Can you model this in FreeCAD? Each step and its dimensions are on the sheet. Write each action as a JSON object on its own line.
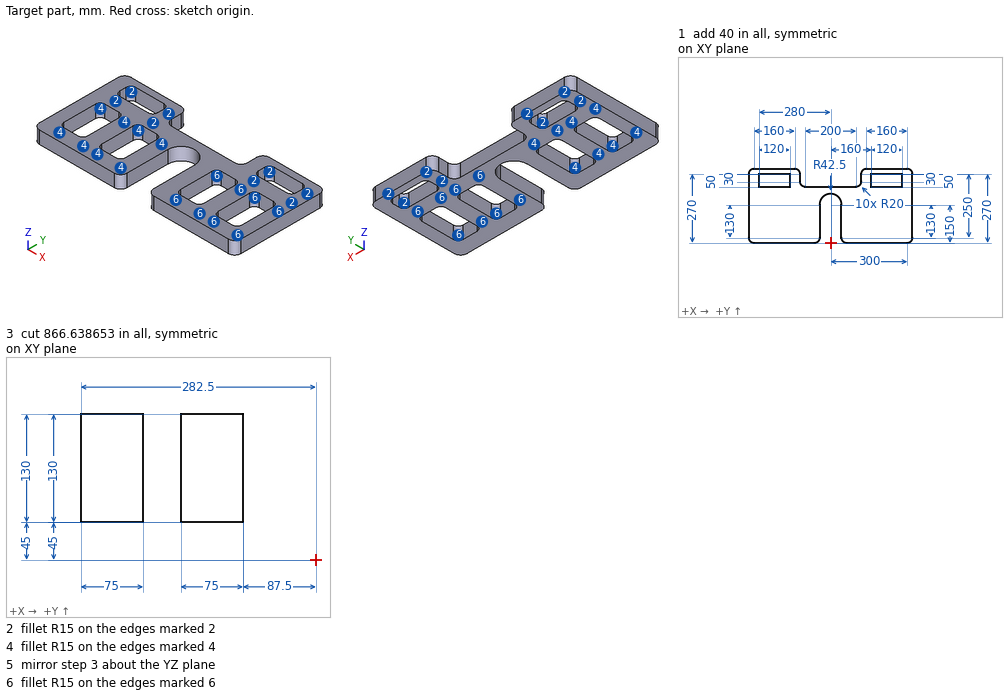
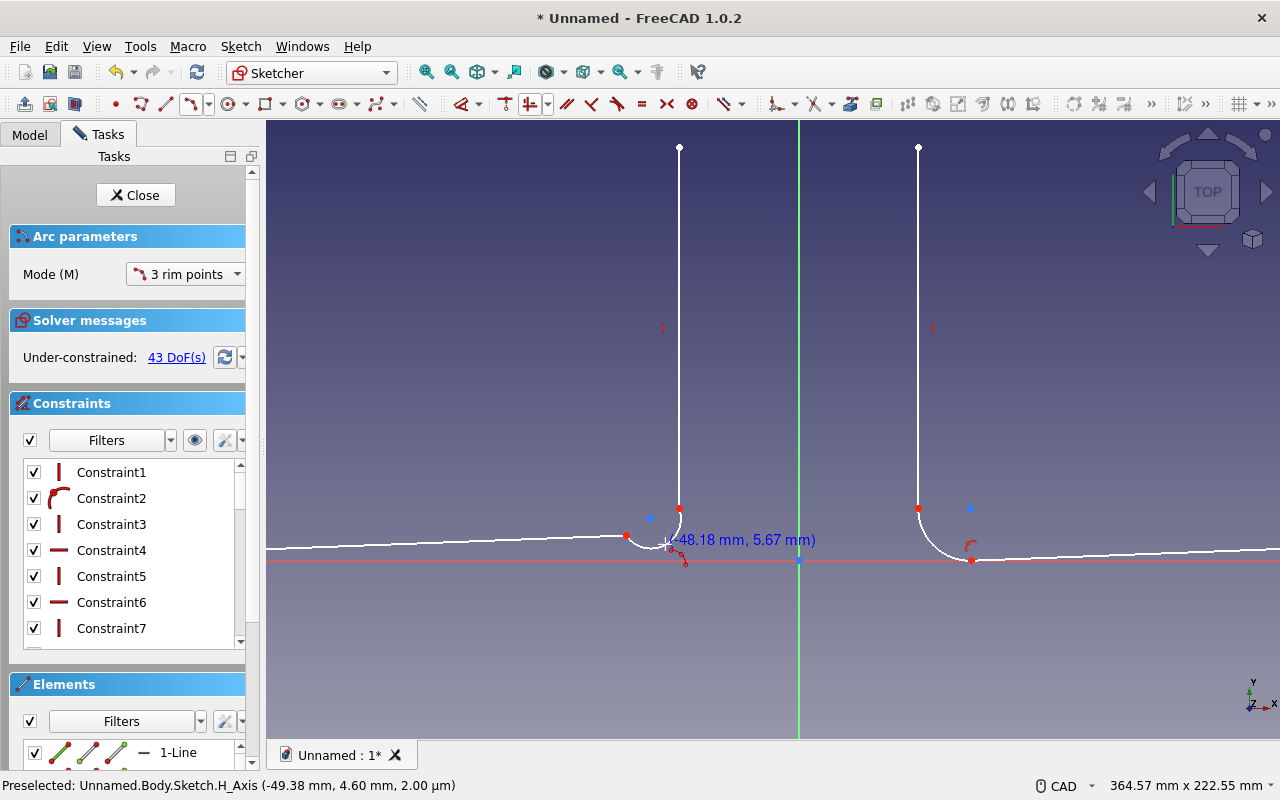
{"action": "scroll", "coordinate": [664, 547], "scroll_direction": "down", "scroll_amount": 6}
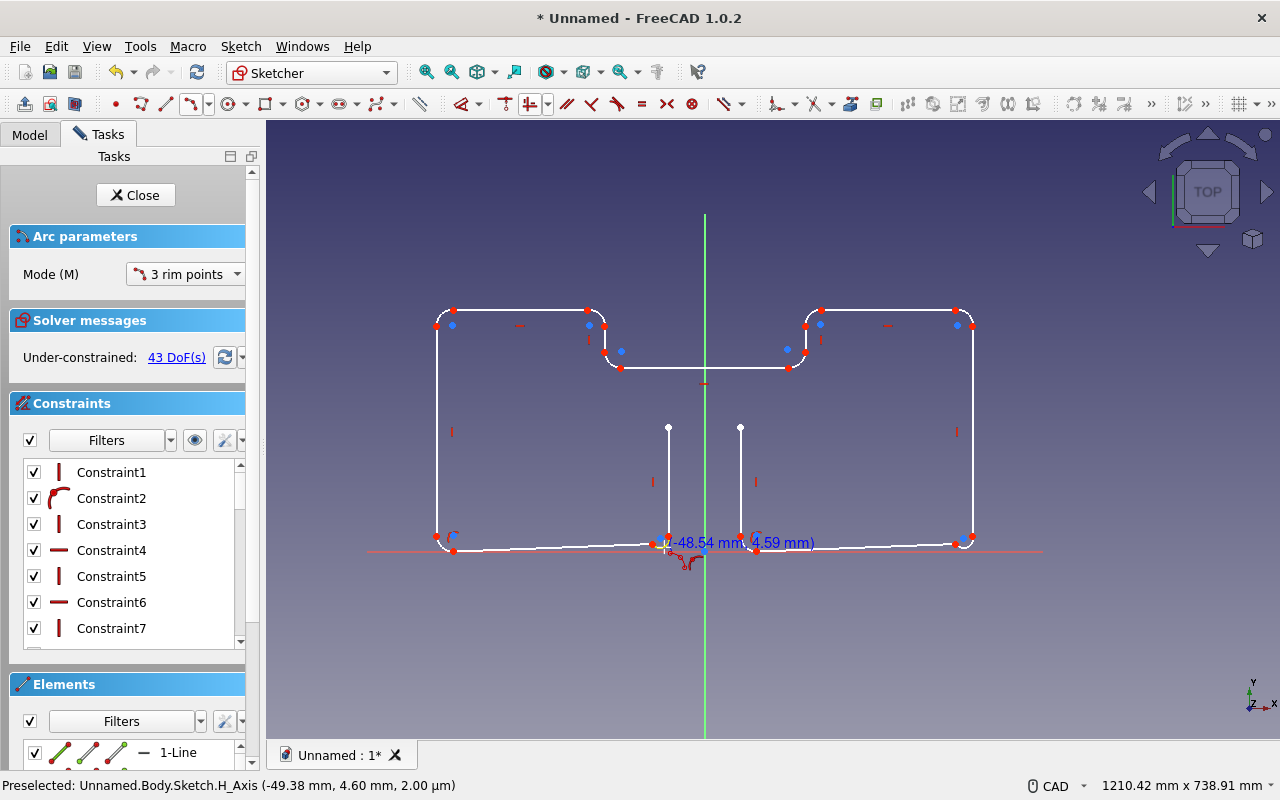
{"action": "left_click", "coordinate": [669, 427]}
{"action": "left_click", "coordinate": [741, 427]}
{"action": "left_click", "coordinate": [726, 397]}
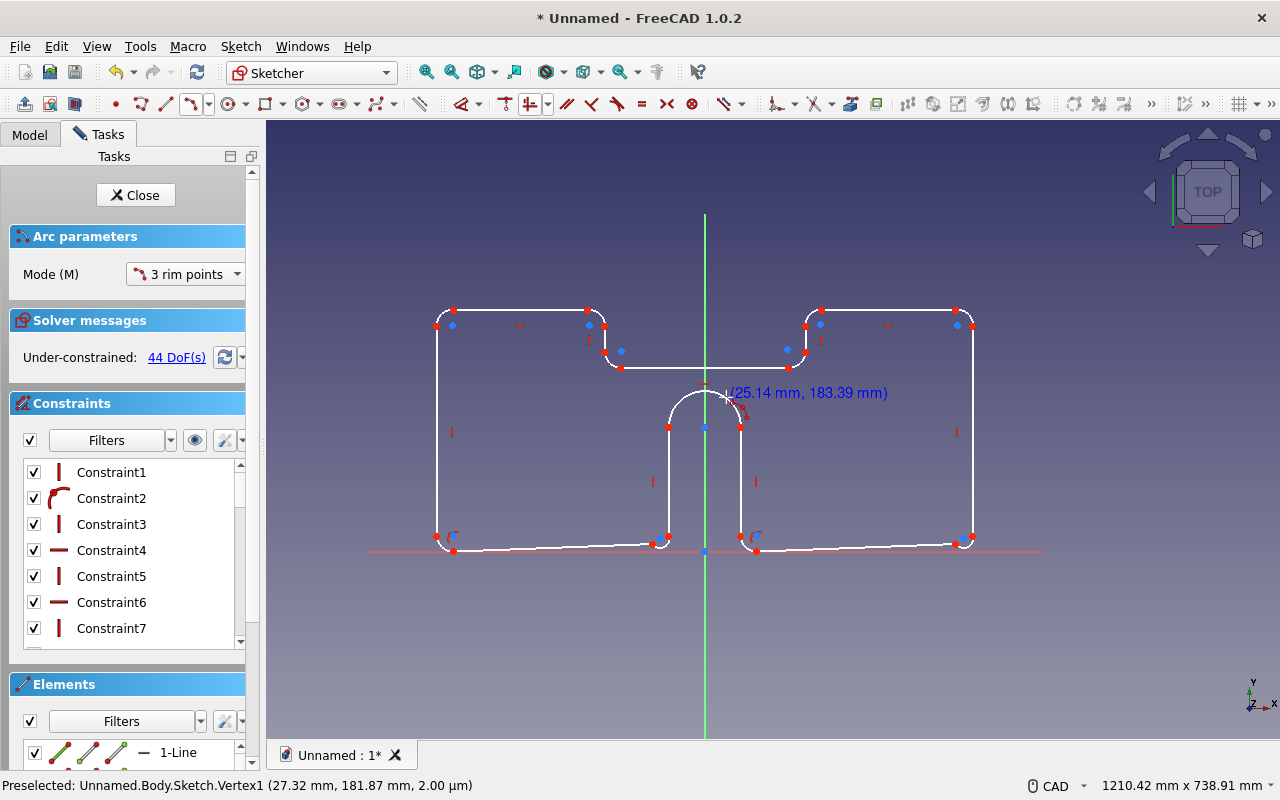
{"action": "left_click", "coordinate": [264, 104]}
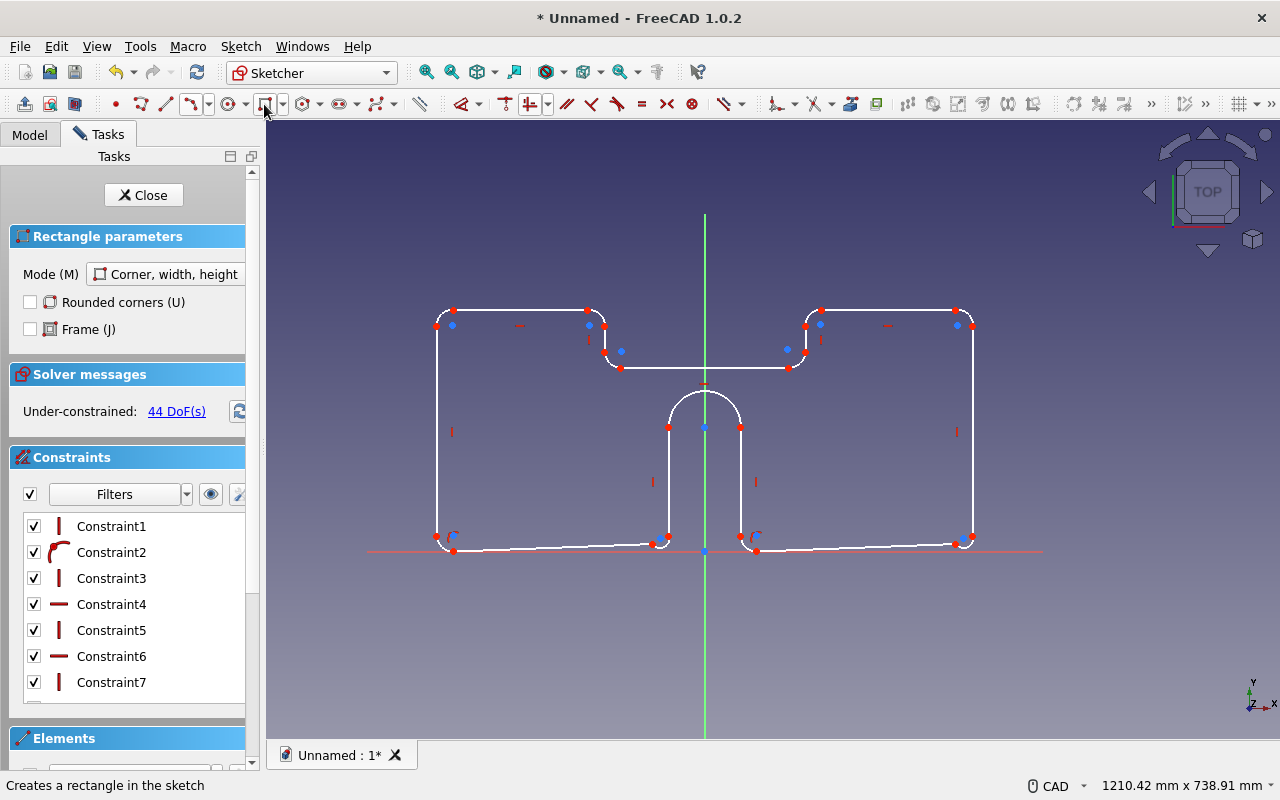
{"action": "left_click", "coordinate": [470, 325]}
{"action": "left_click", "coordinate": [571, 367]}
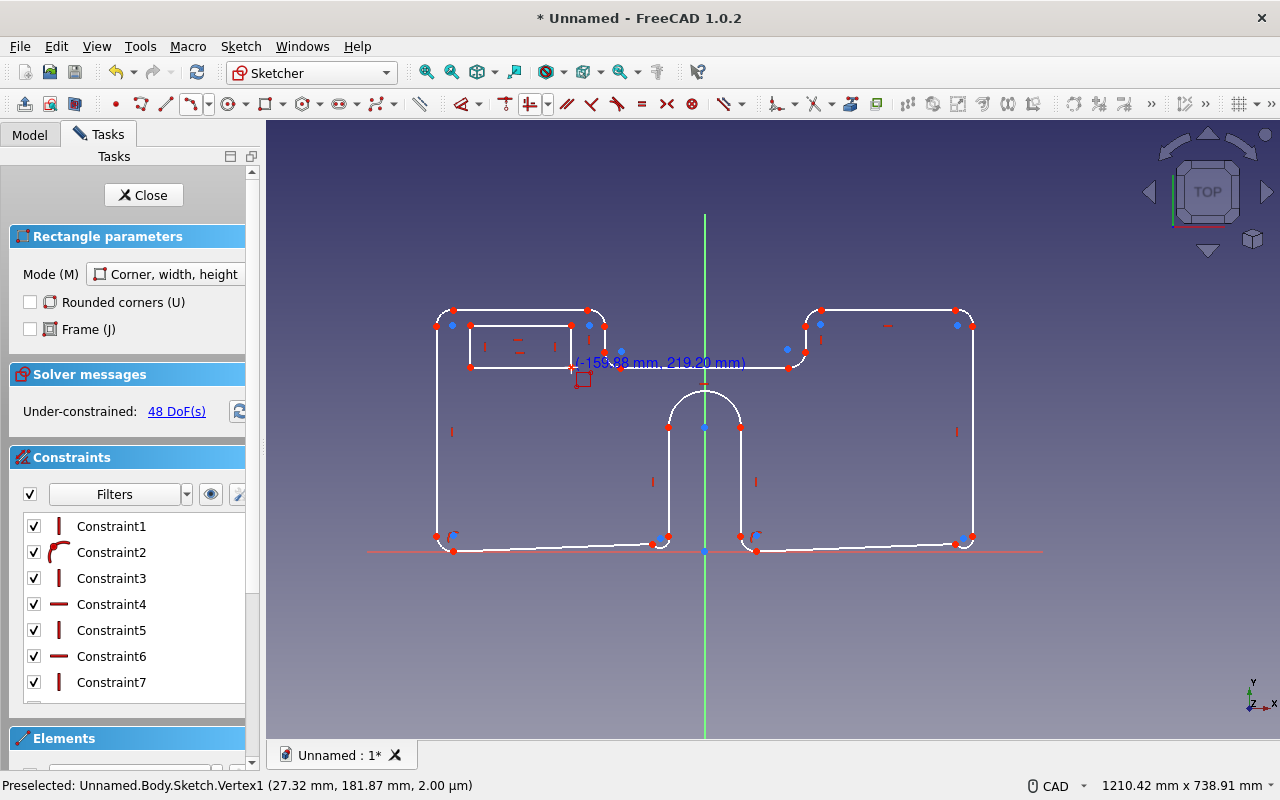
{"action": "left_click", "coordinate": [839, 325]}
{"action": "left_click", "coordinate": [940, 367]}
{"action": "key", "text": "Escape"}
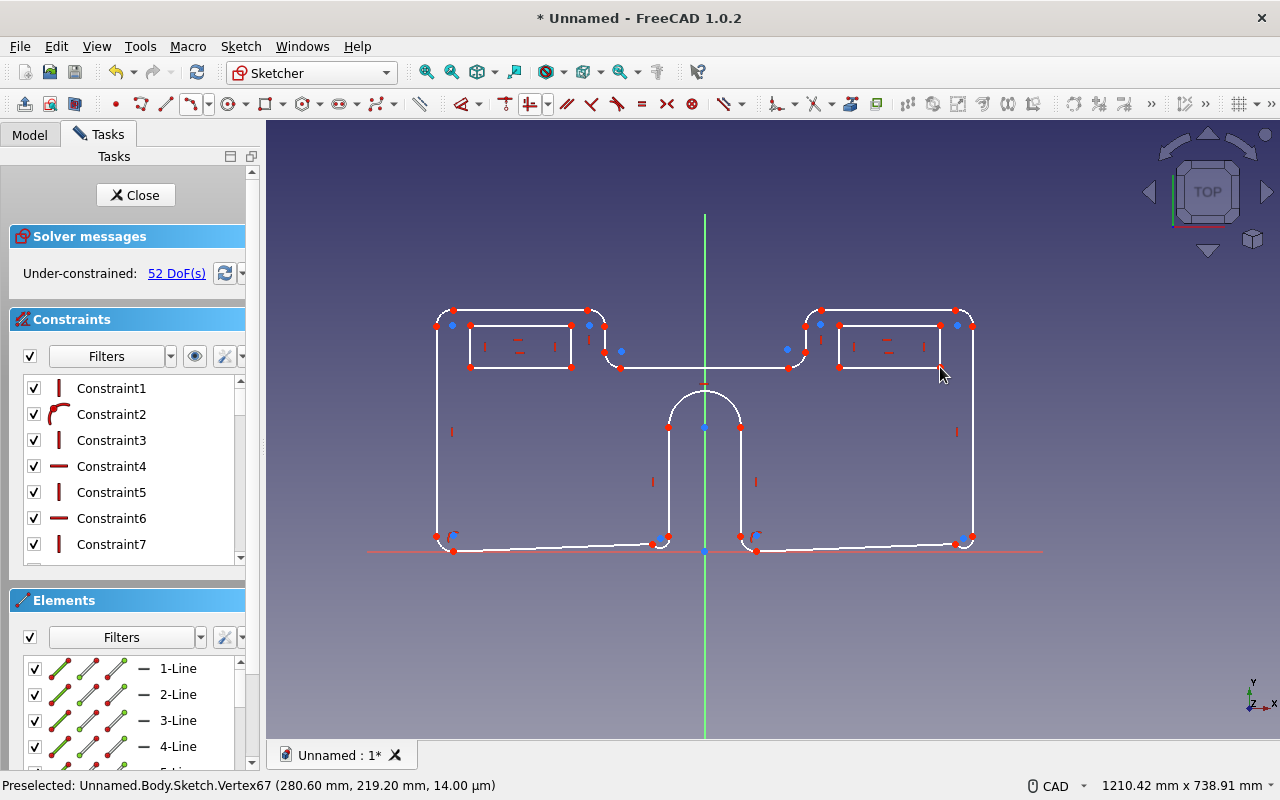
{"action": "left_click", "coordinate": [741, 460]}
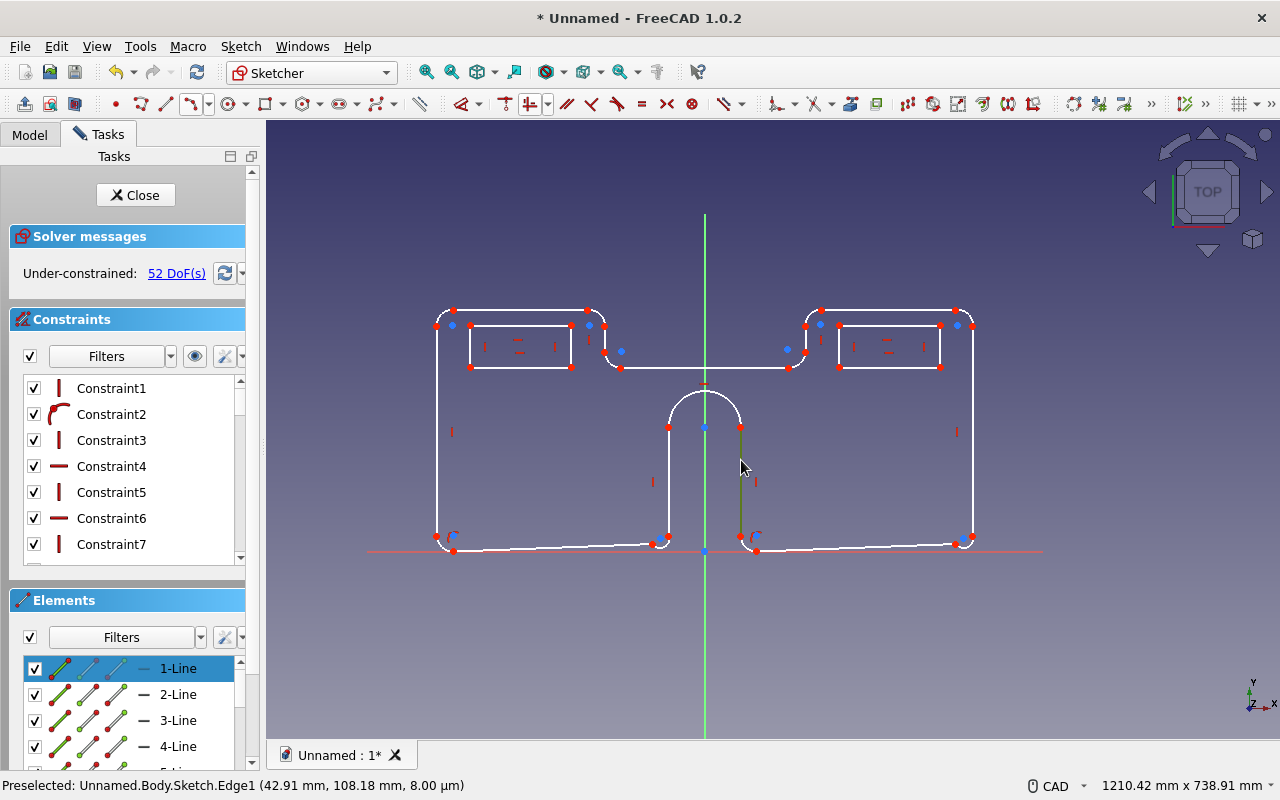
{"action": "scroll", "coordinate": [743, 543], "scroll_direction": "up", "scroll_amount": 4}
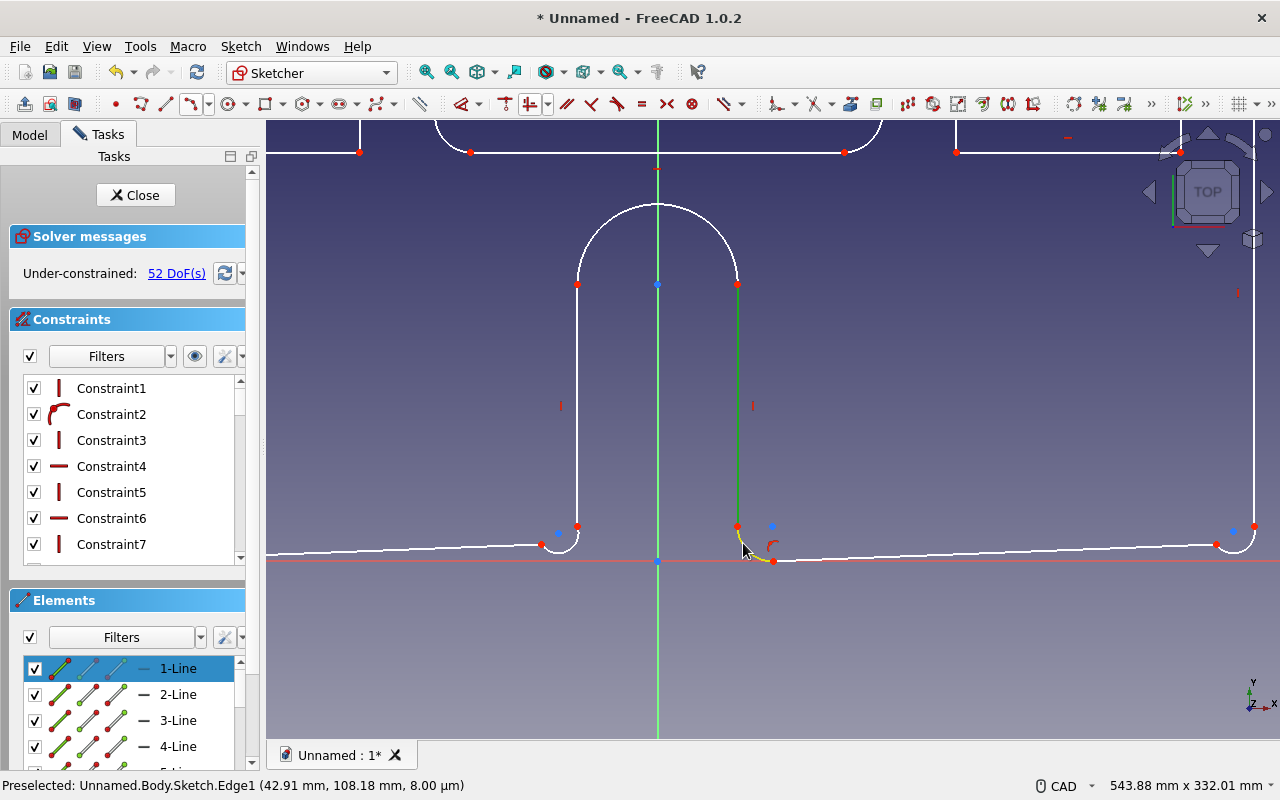
{"action": "left_click", "coordinate": [742, 543]}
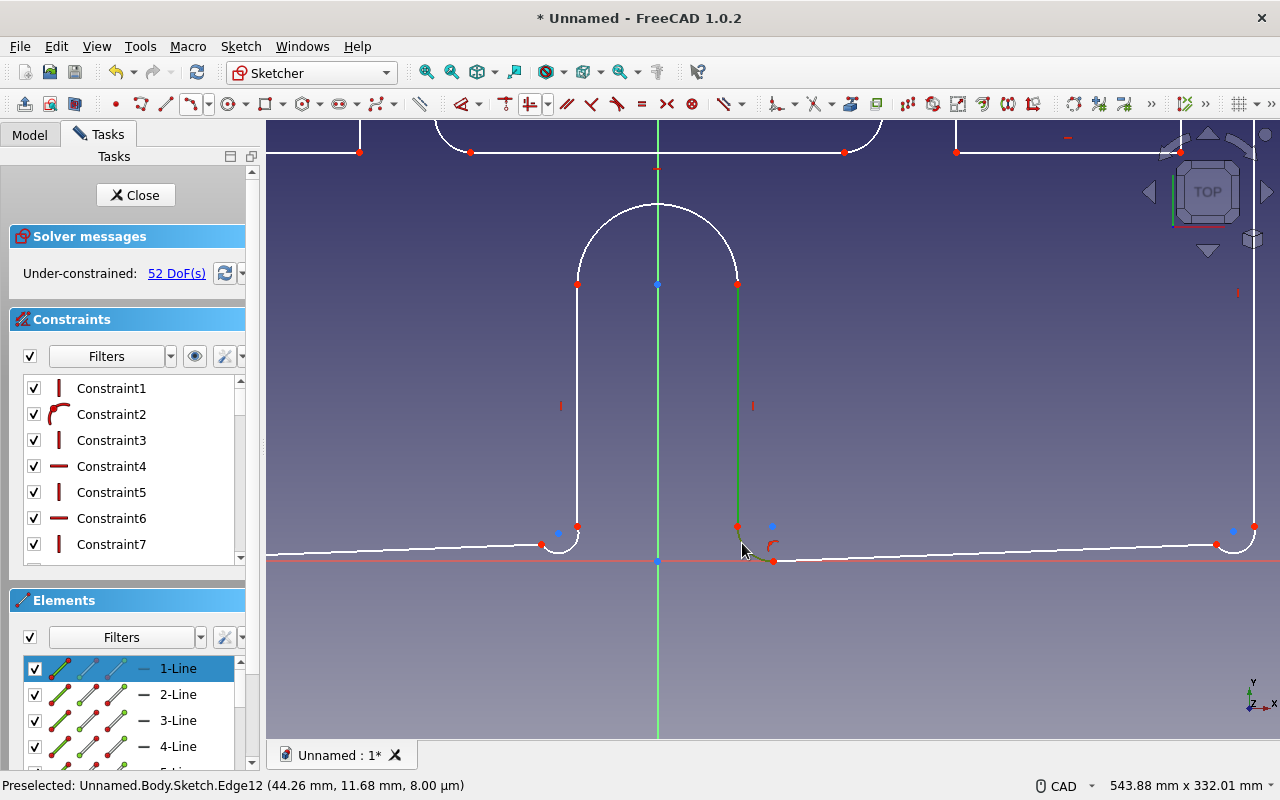
{"action": "left_click", "coordinate": [617, 104]}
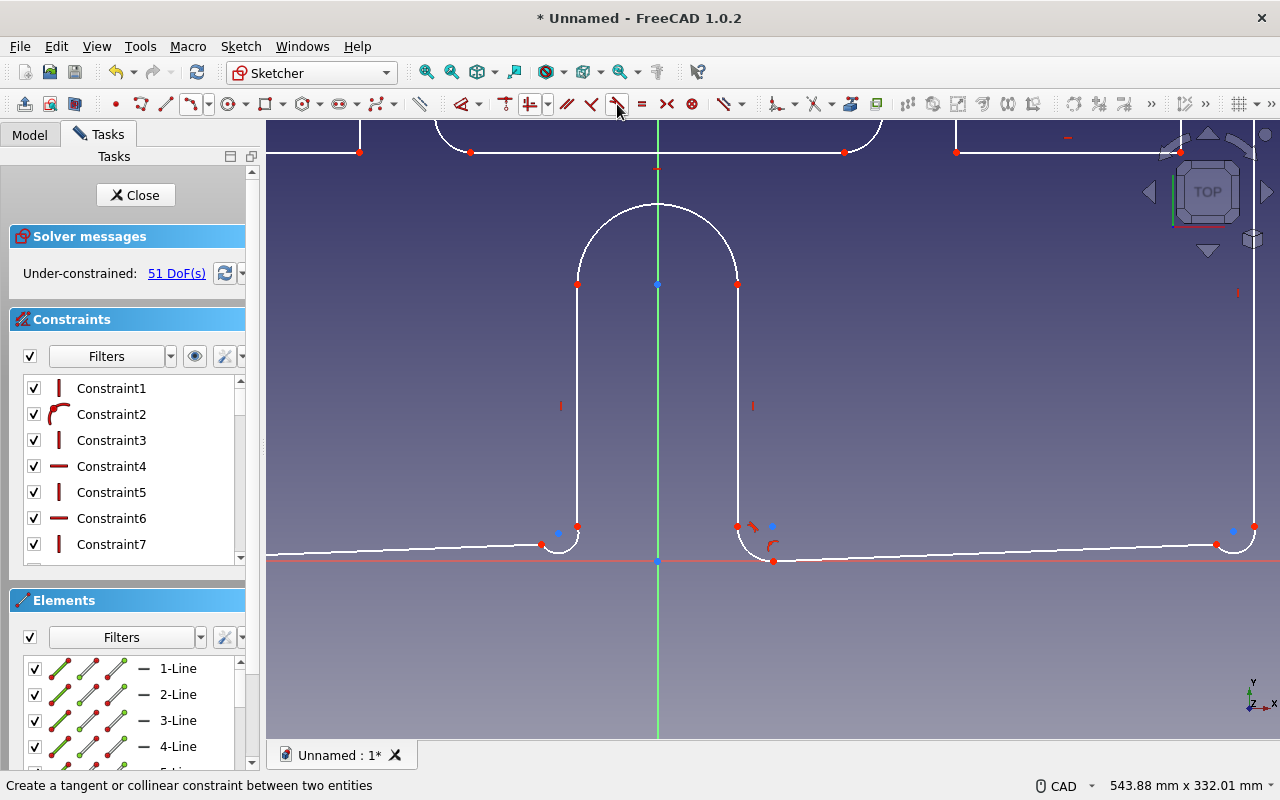
{"action": "left_click", "coordinate": [1083, 550]}